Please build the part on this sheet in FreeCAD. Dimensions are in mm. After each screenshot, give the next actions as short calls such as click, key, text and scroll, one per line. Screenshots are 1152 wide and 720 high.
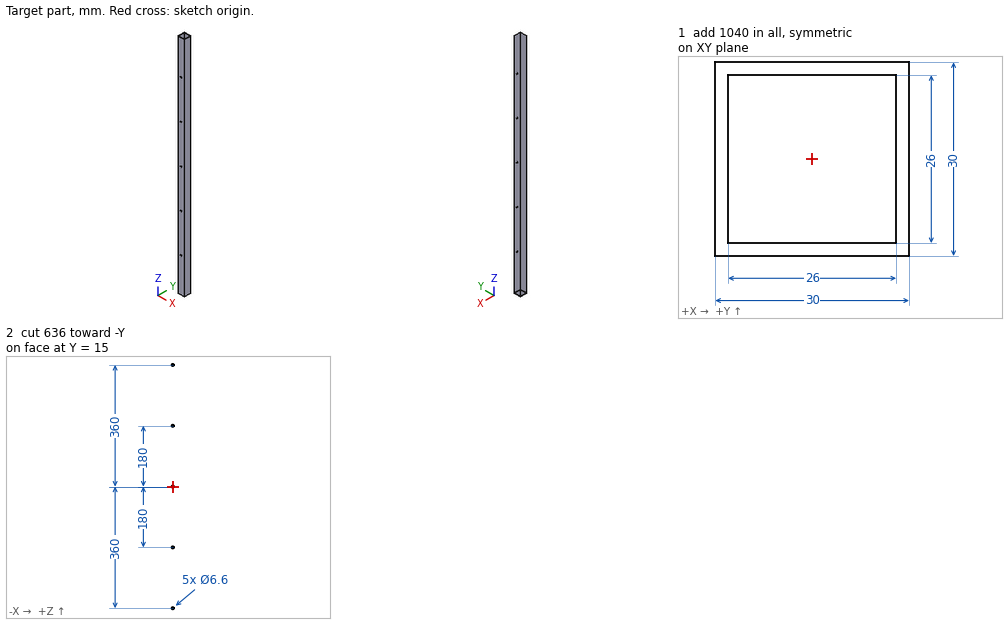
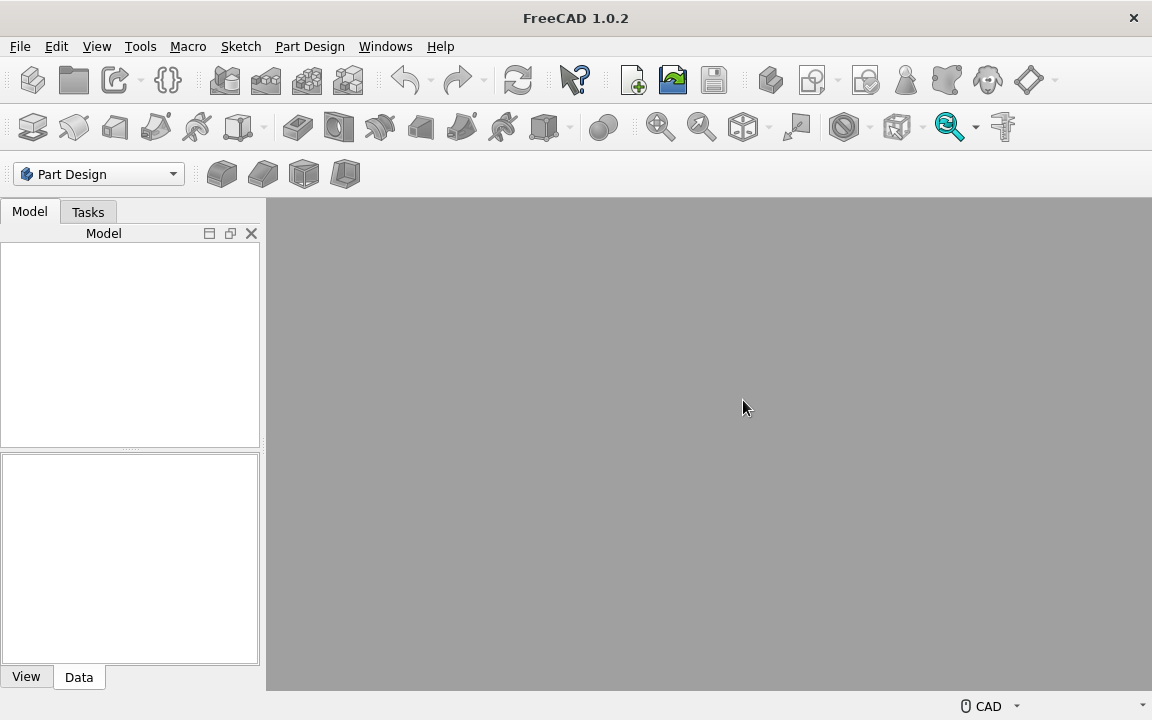
click(632, 80)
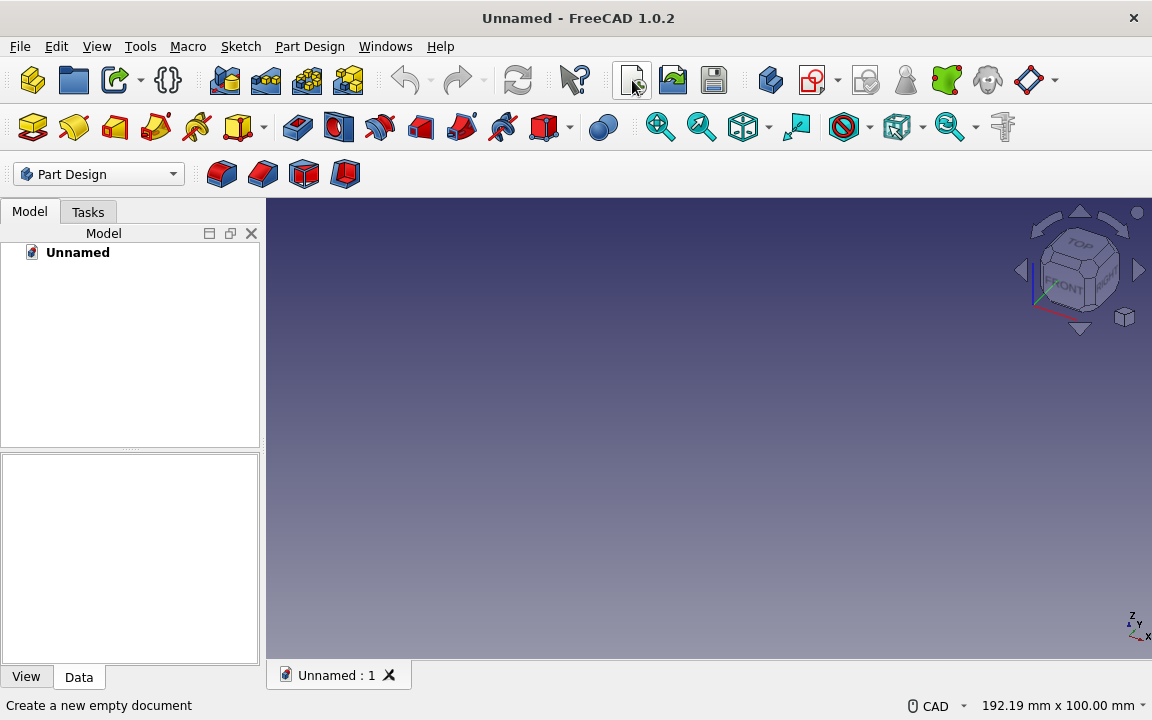
click(812, 80)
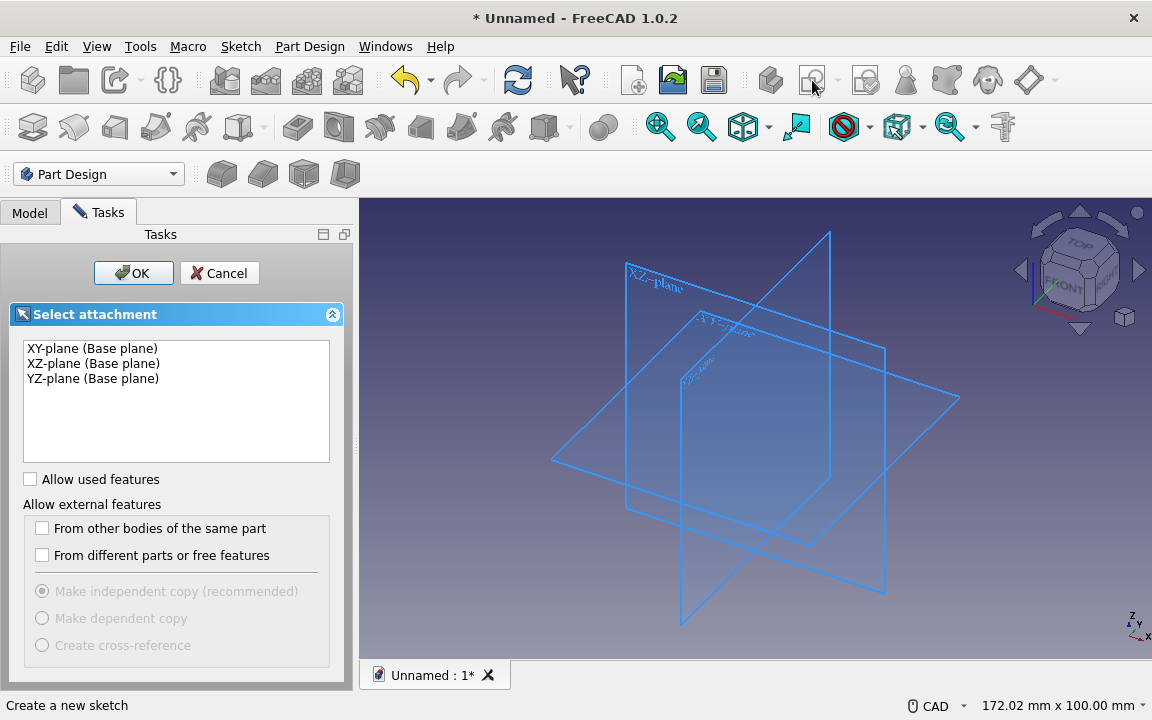
click(84, 348)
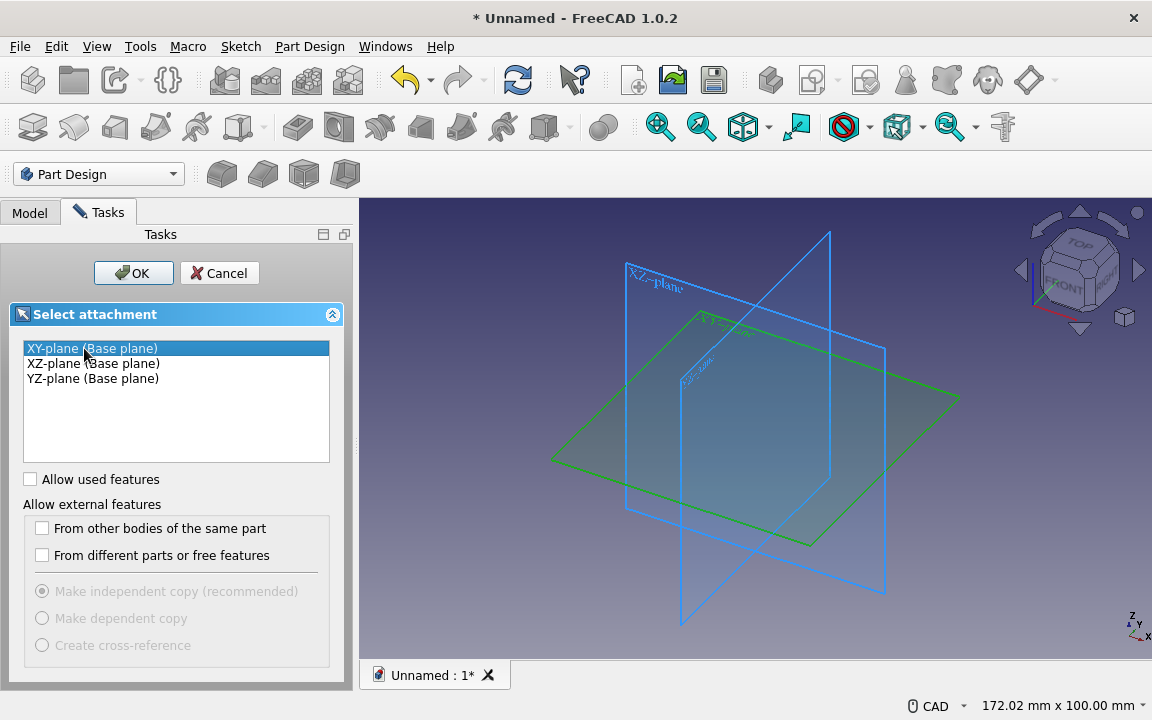
click(134, 273)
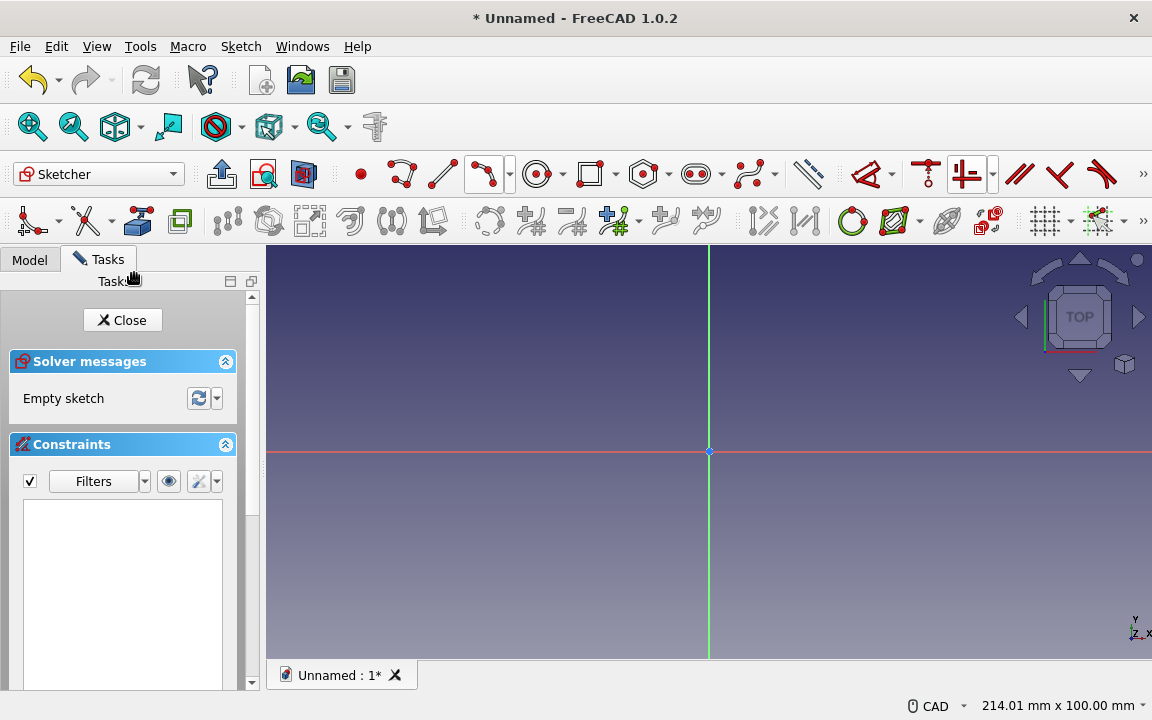
scroll(765, 452, up, 4)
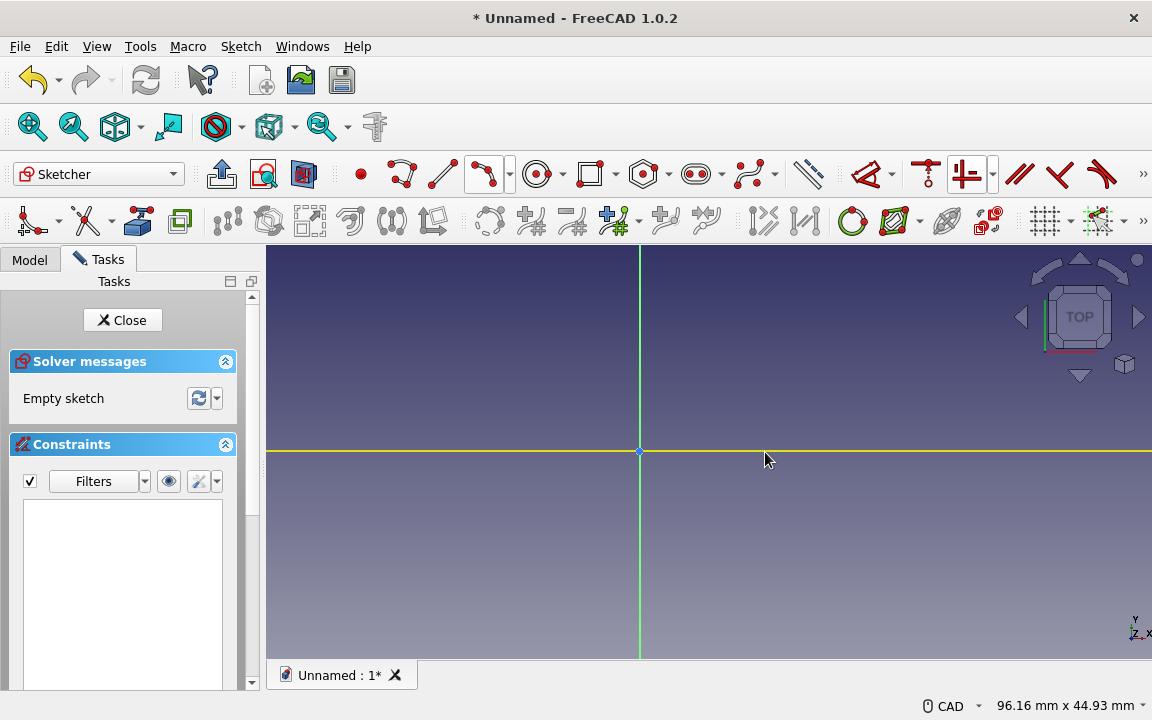
key(g)
key(v)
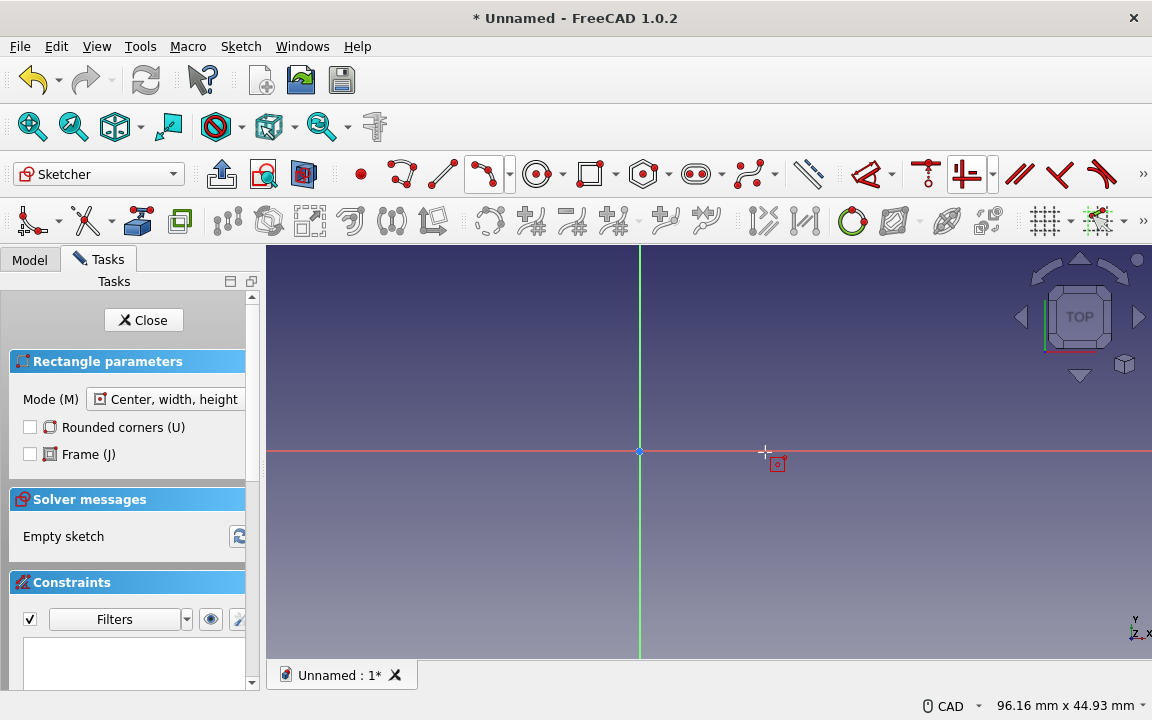
click(640, 451)
move(778, 313)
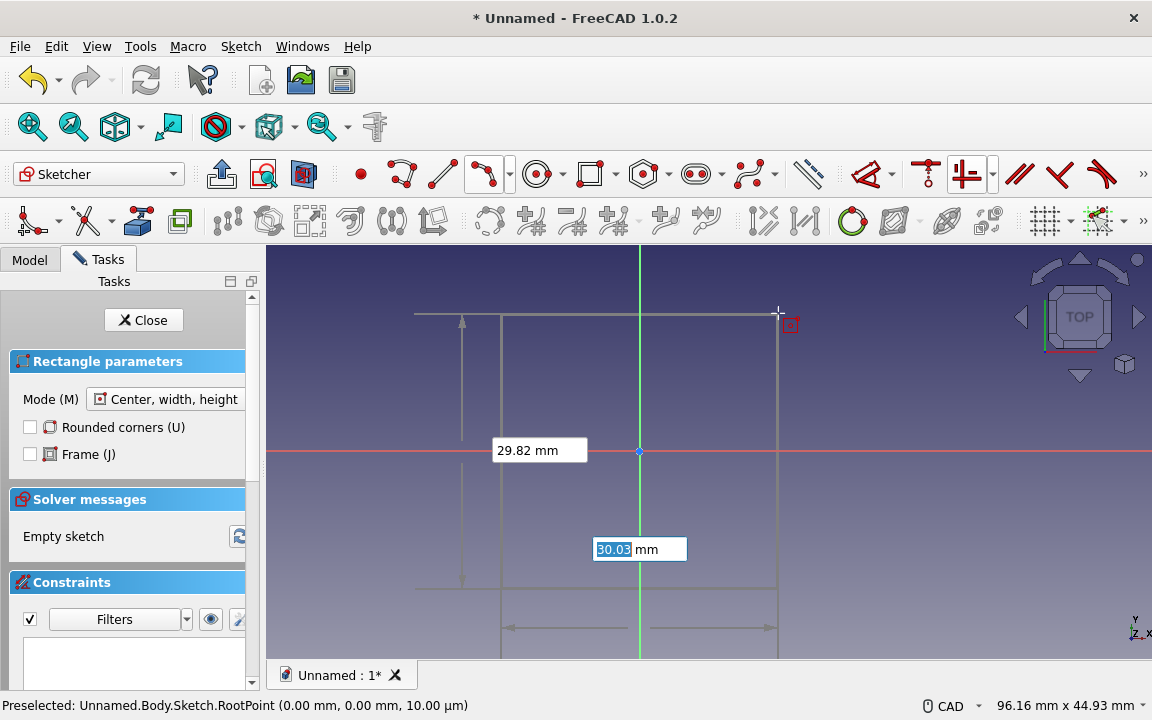
text(30)
key(Tab)
text(30)
key(Return)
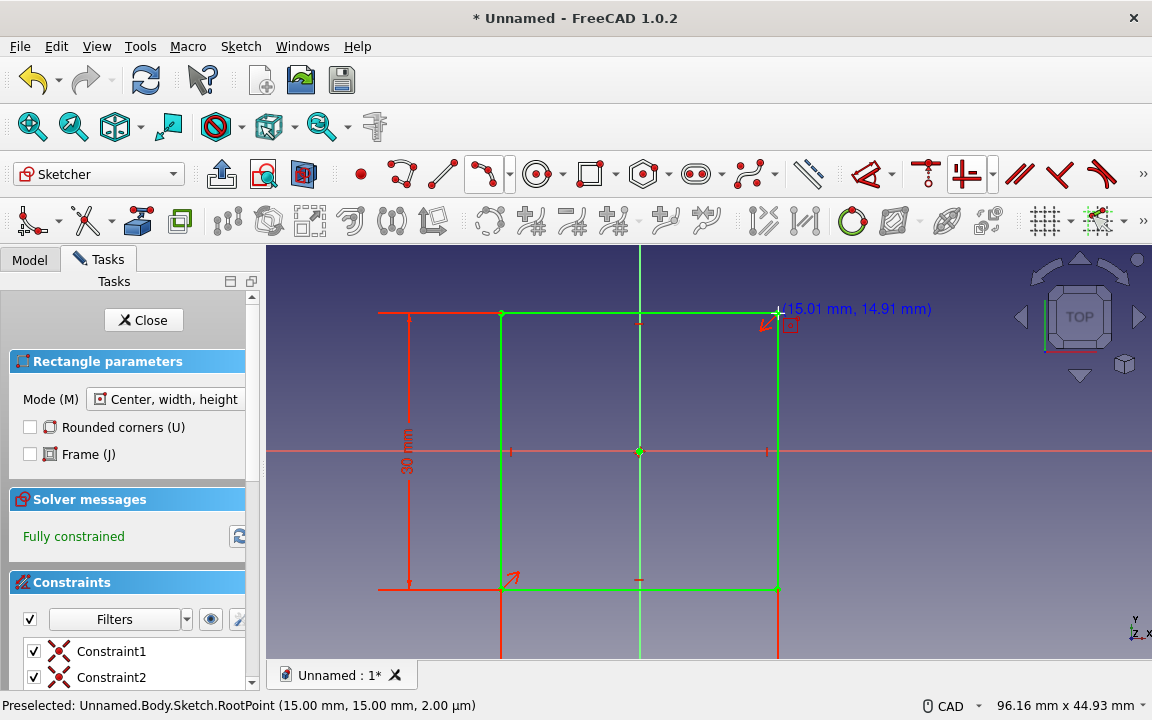
click(640, 451)
move(759, 332)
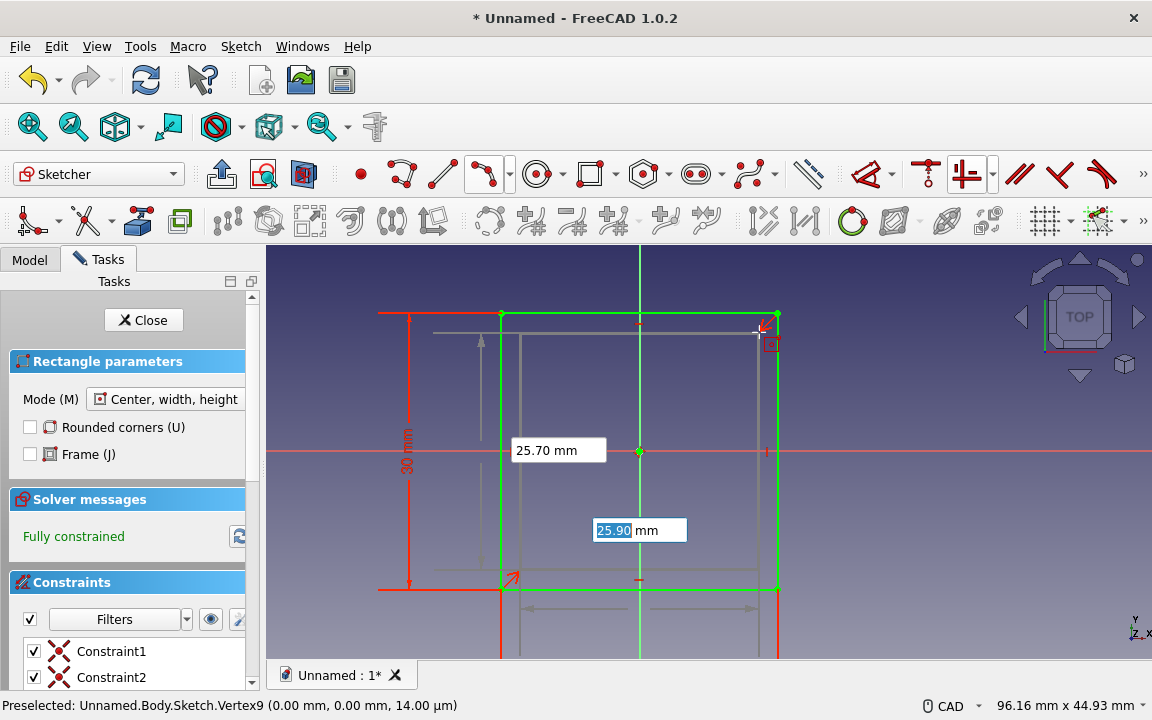
text(26)
key(Tab)
text(26)
key(Return)
key(Escape)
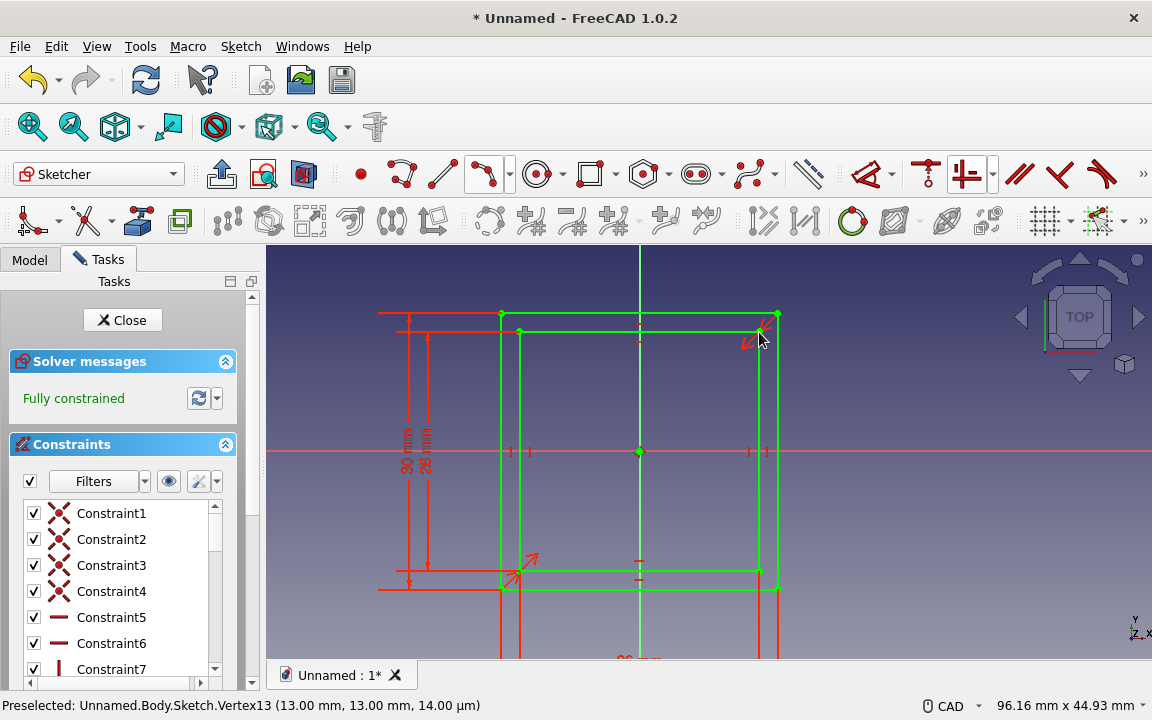
click(123, 320)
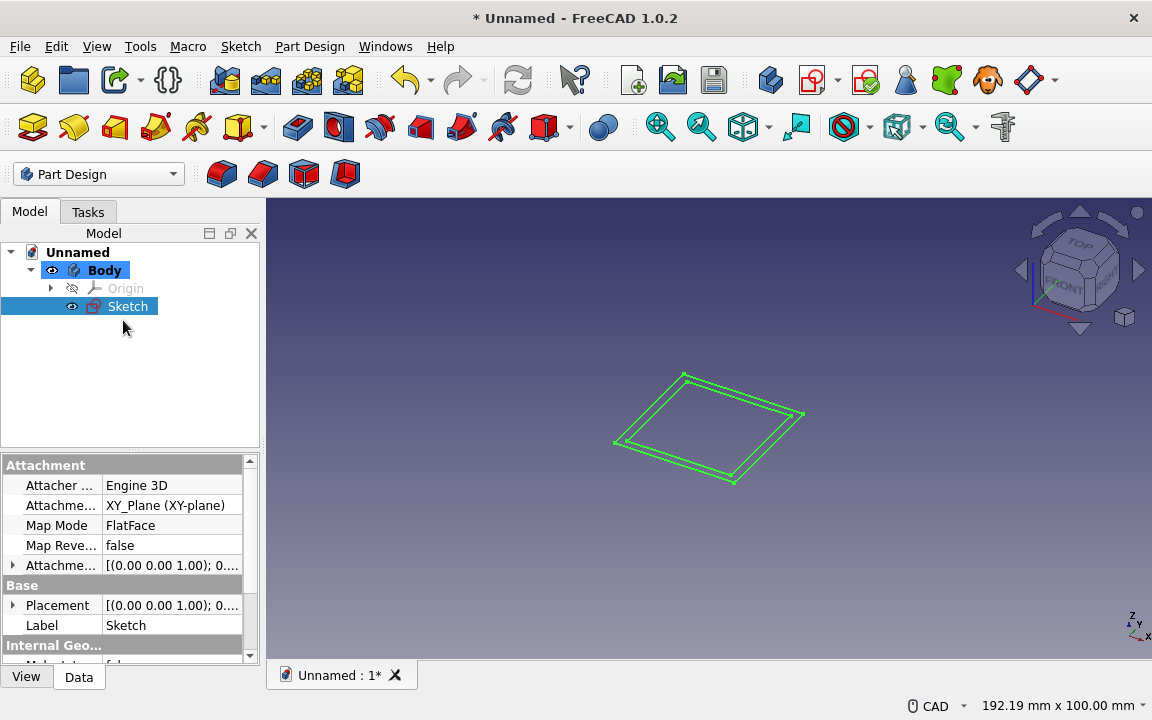
click(33, 128)